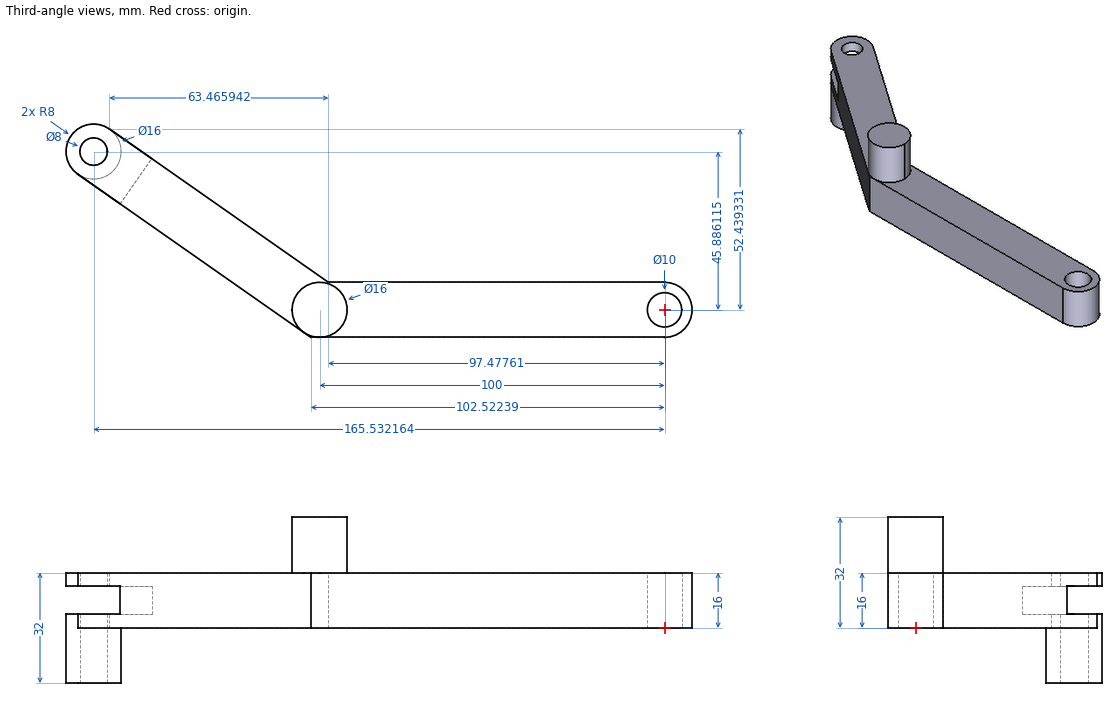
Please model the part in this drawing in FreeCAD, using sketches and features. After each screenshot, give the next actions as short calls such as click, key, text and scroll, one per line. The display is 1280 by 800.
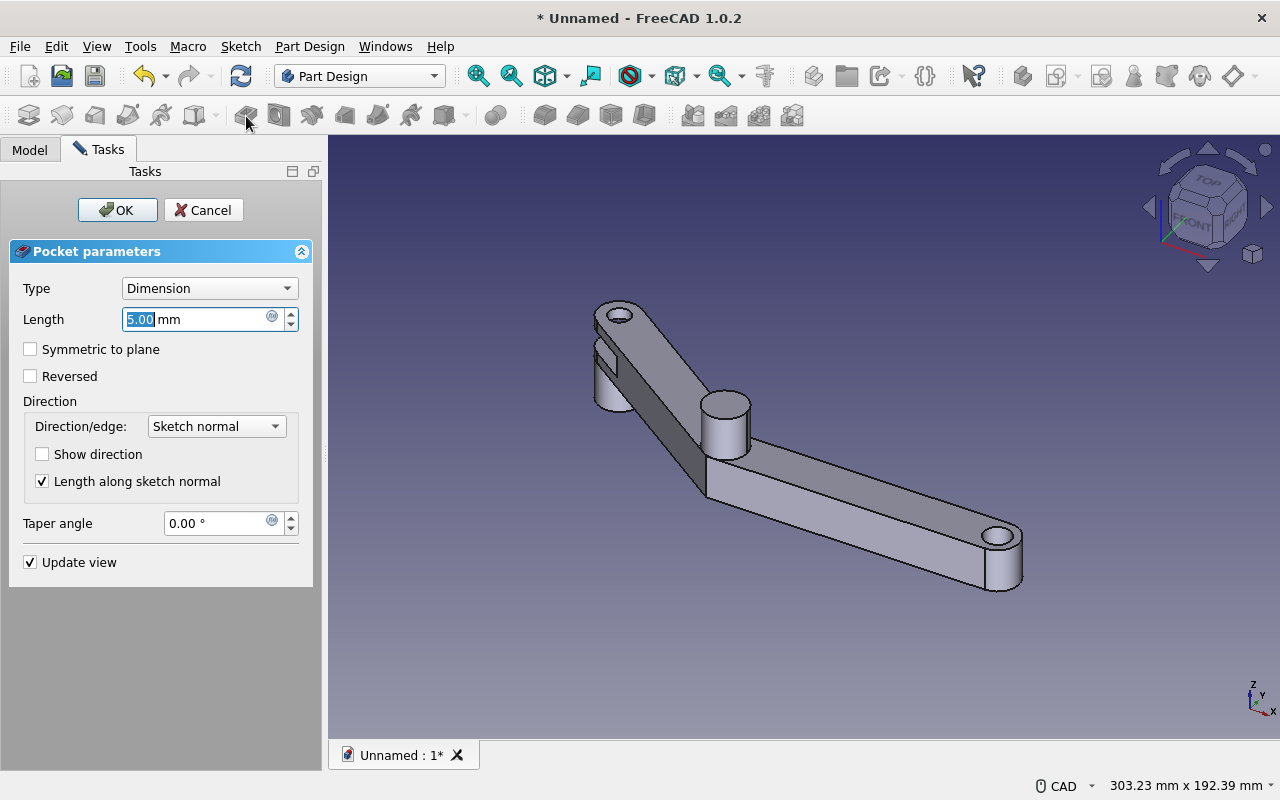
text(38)
key(Tab)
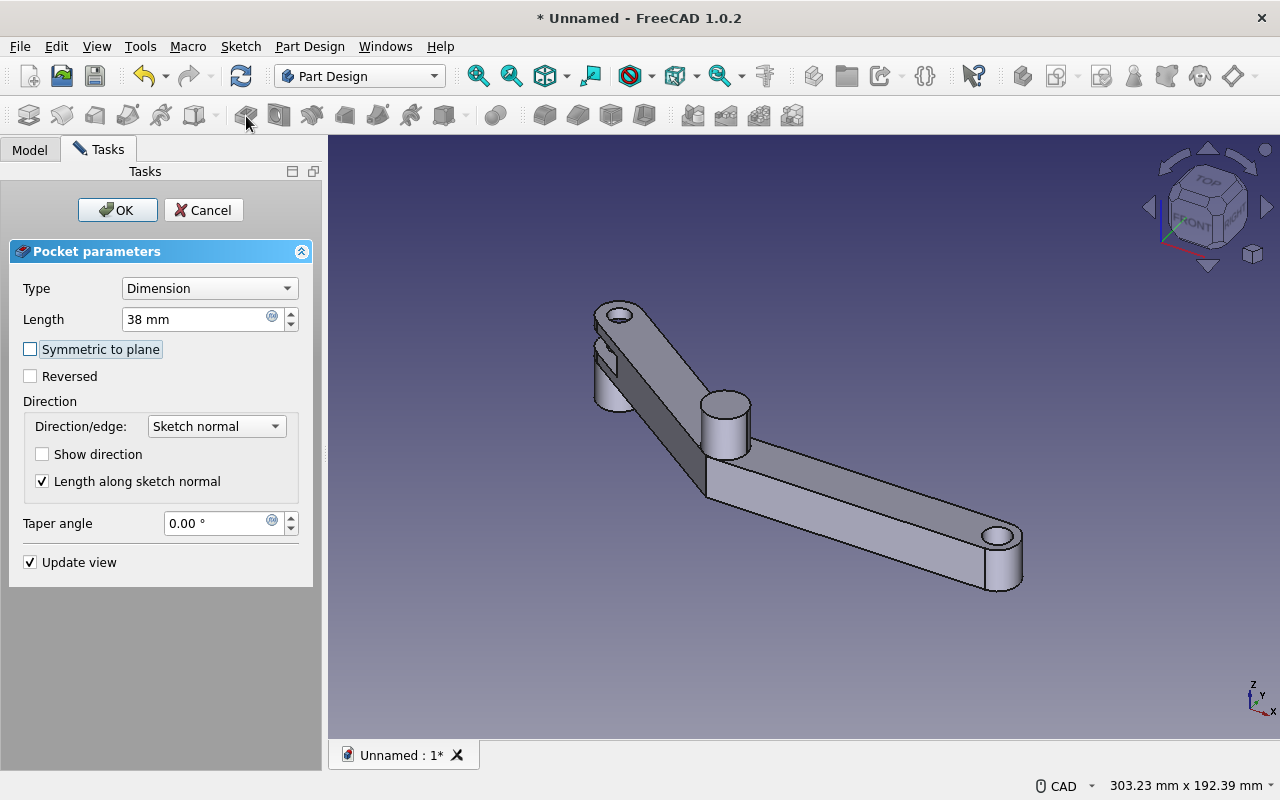
click(118, 210)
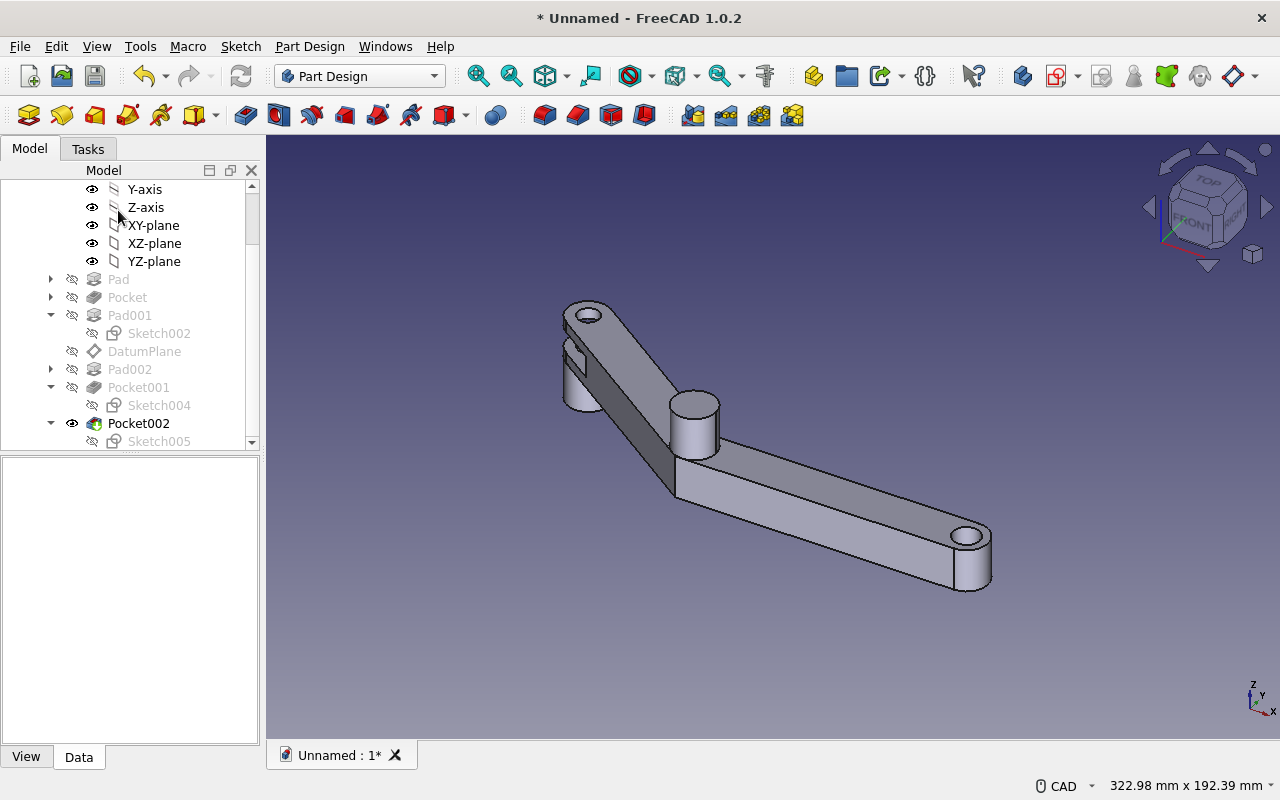
key(0)